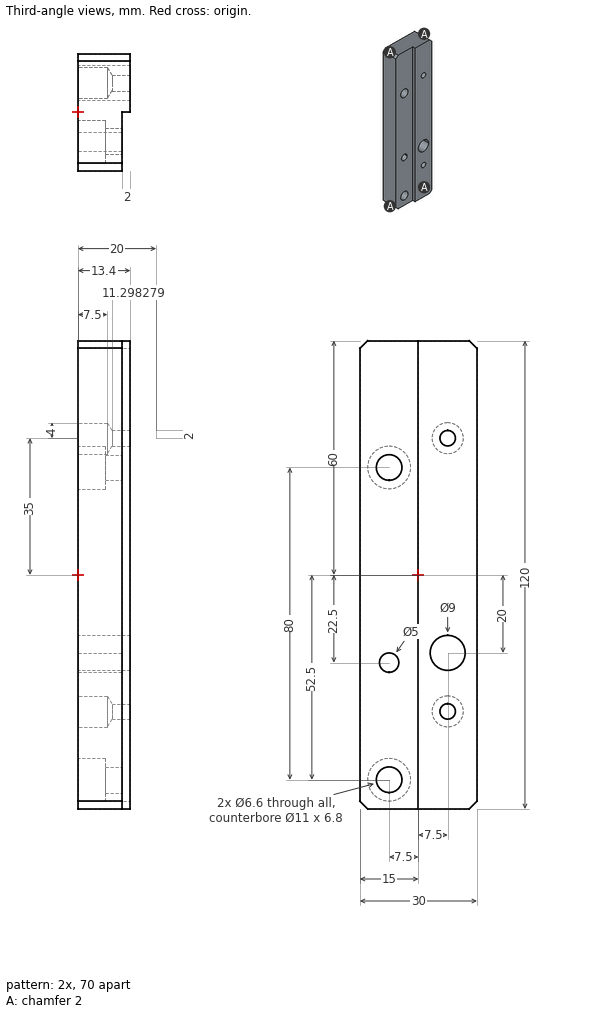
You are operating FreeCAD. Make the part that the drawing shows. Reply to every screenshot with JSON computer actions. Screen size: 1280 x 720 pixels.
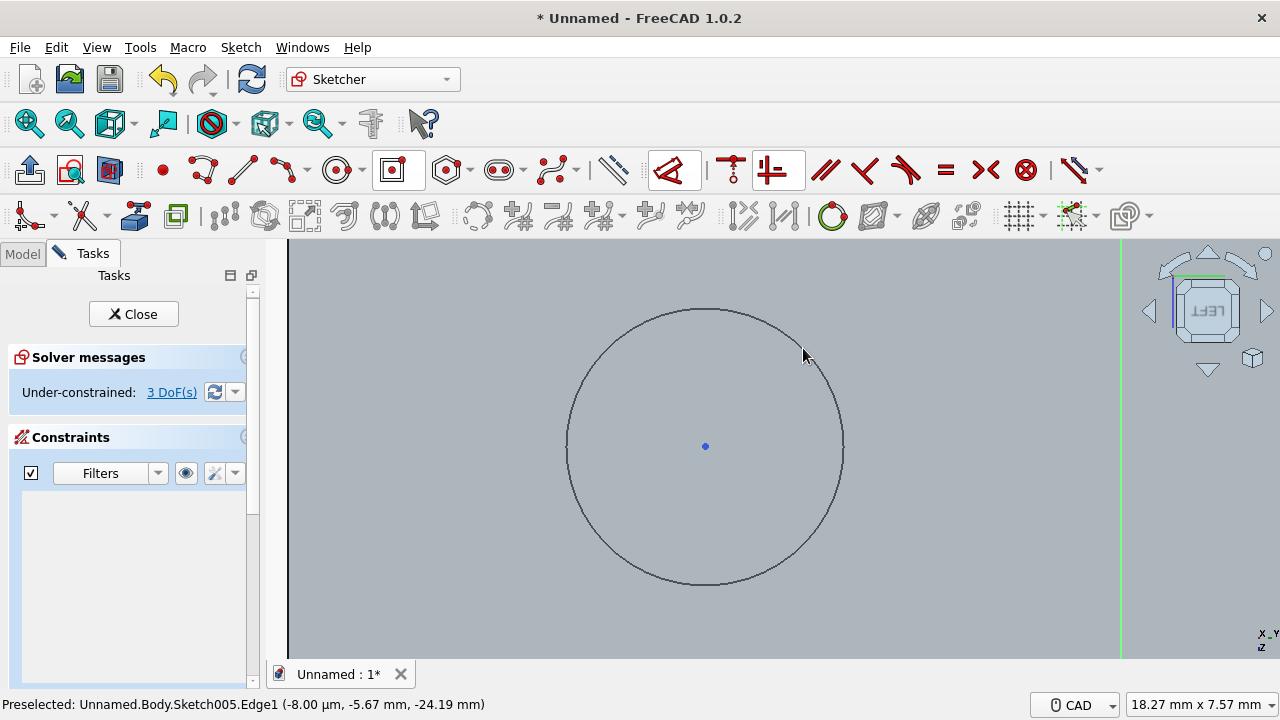
{"action": "left_click", "coordinate": [803, 349]}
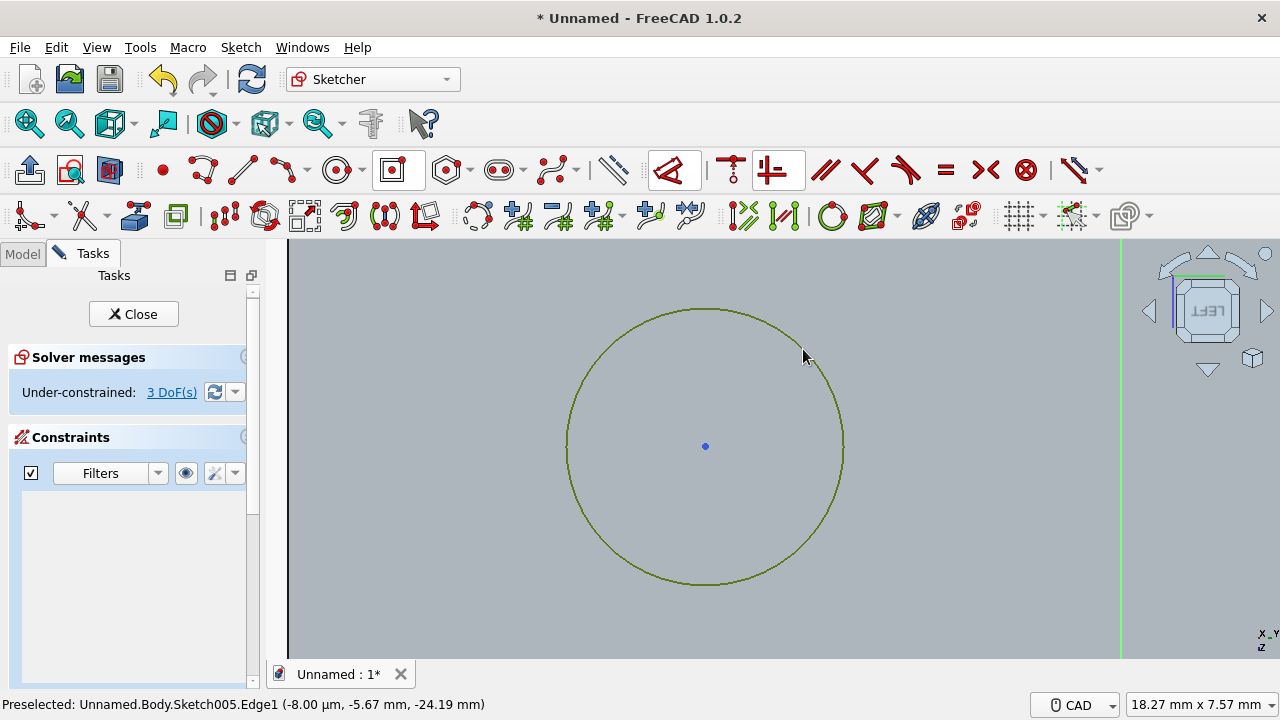
{"action": "left_click", "coordinate": [696, 170]}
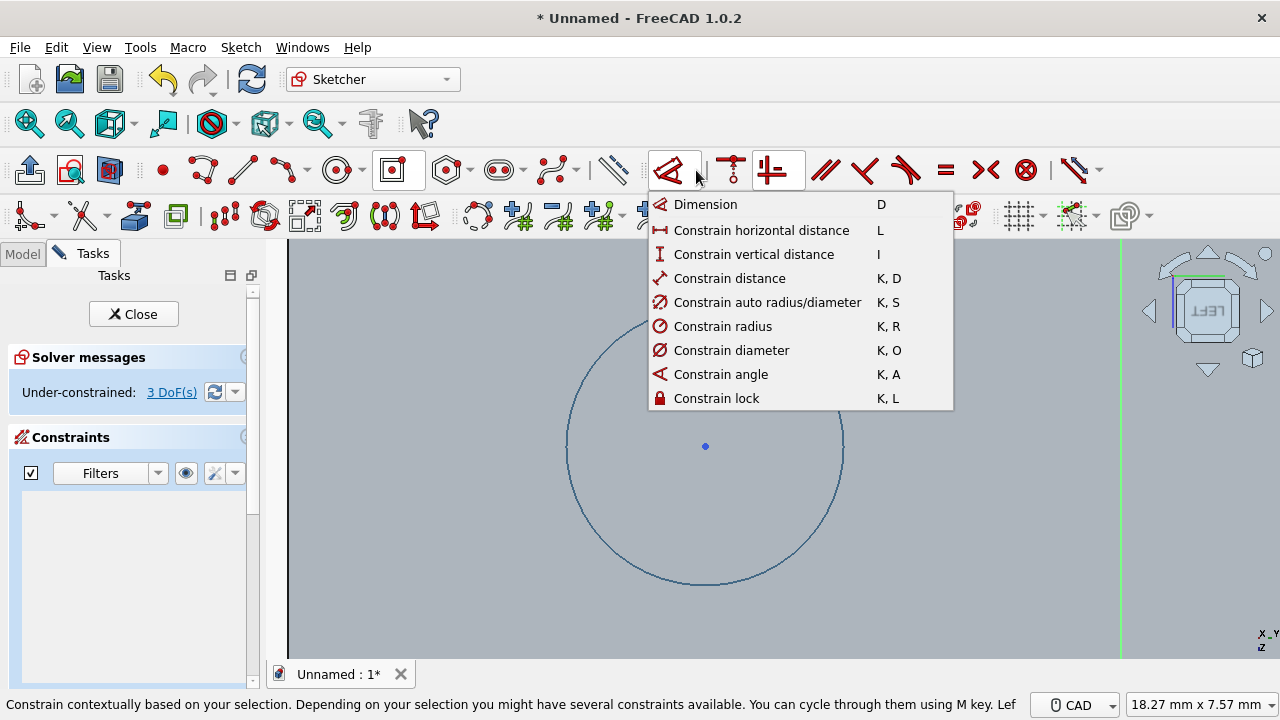
{"action": "left_click", "coordinate": [801, 350]}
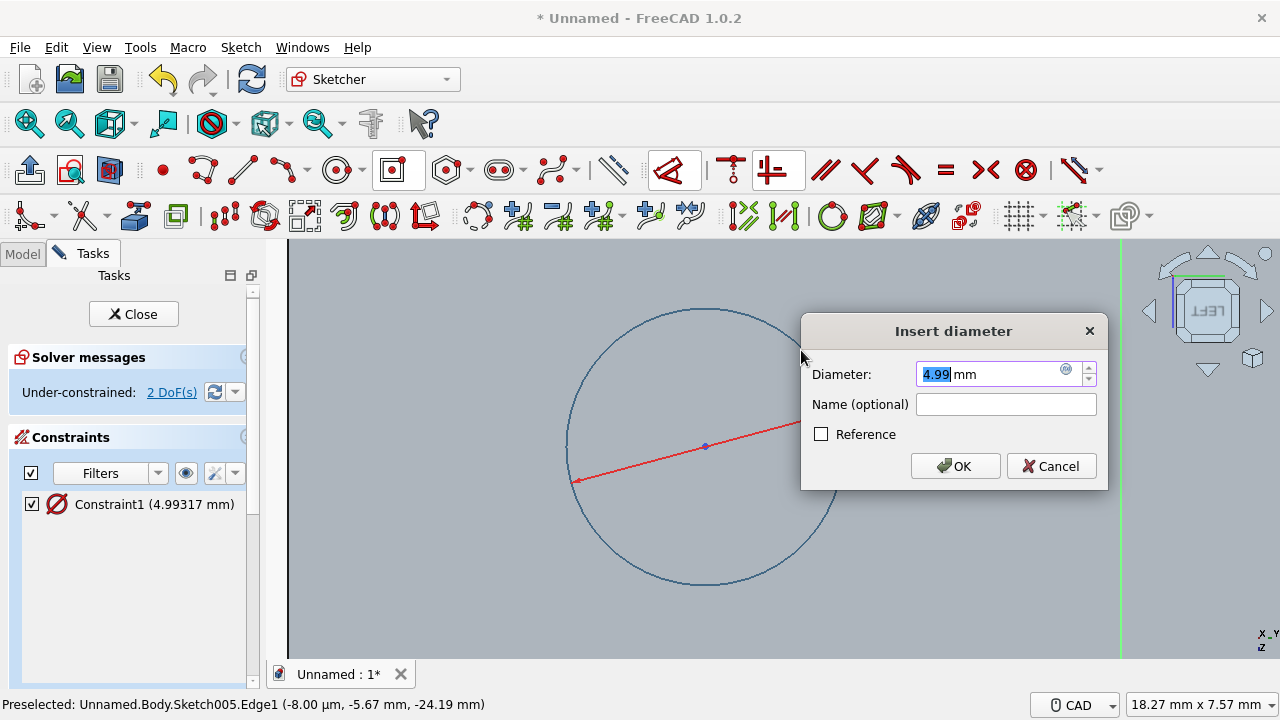
{"action": "type", "text": "5"}
{"action": "key", "text": "Return"}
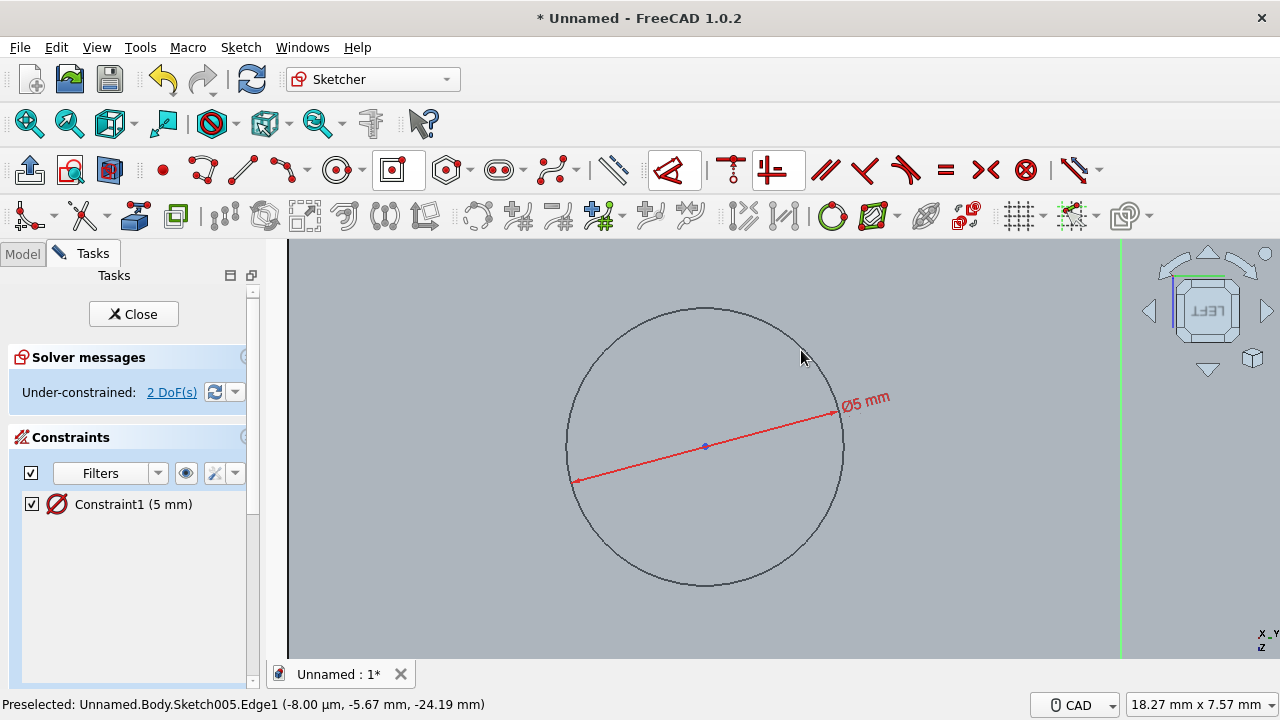
{"action": "left_click", "coordinate": [705, 447]}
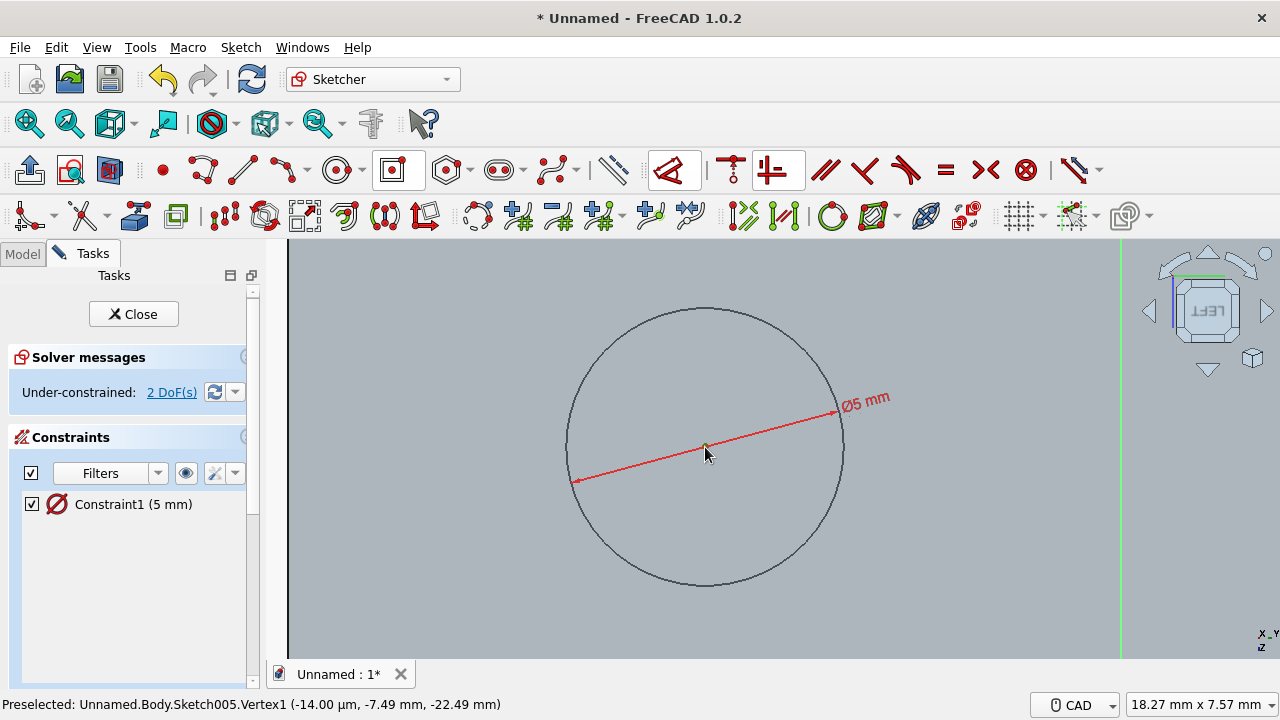
{"action": "key", "text": "l"}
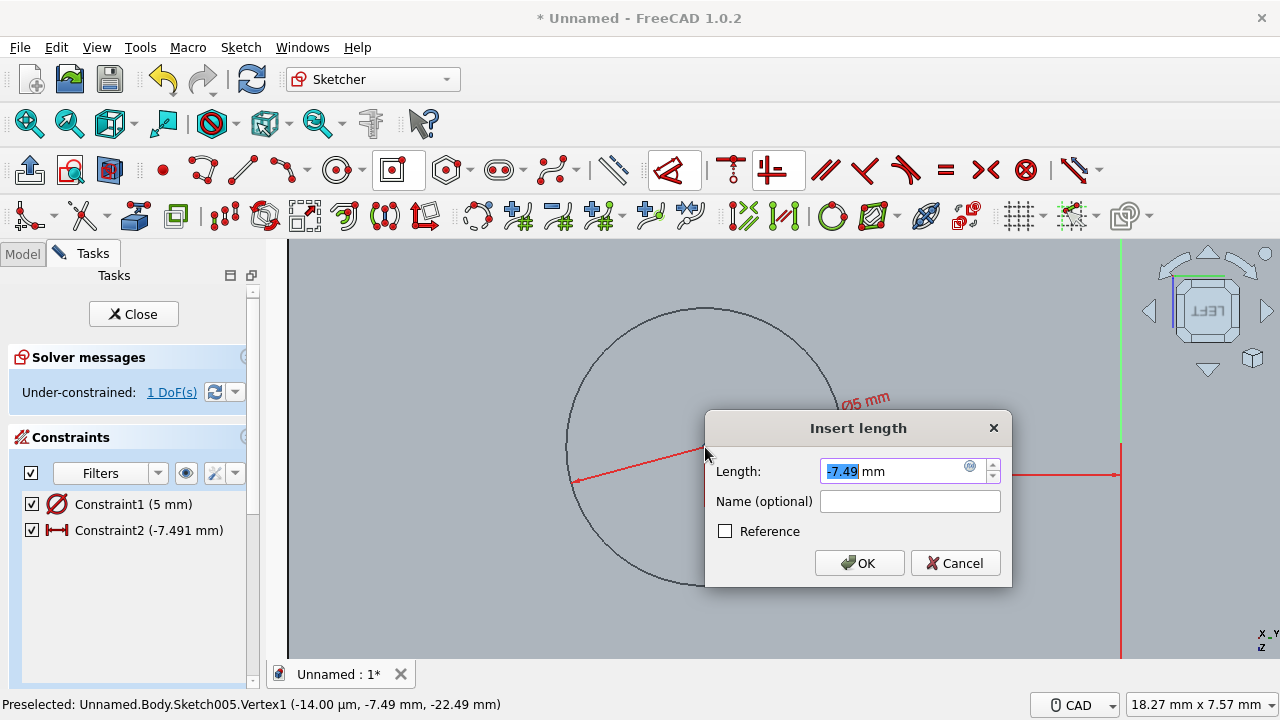
{"action": "type", "text": "-7.5"}
{"action": "key", "text": "Return"}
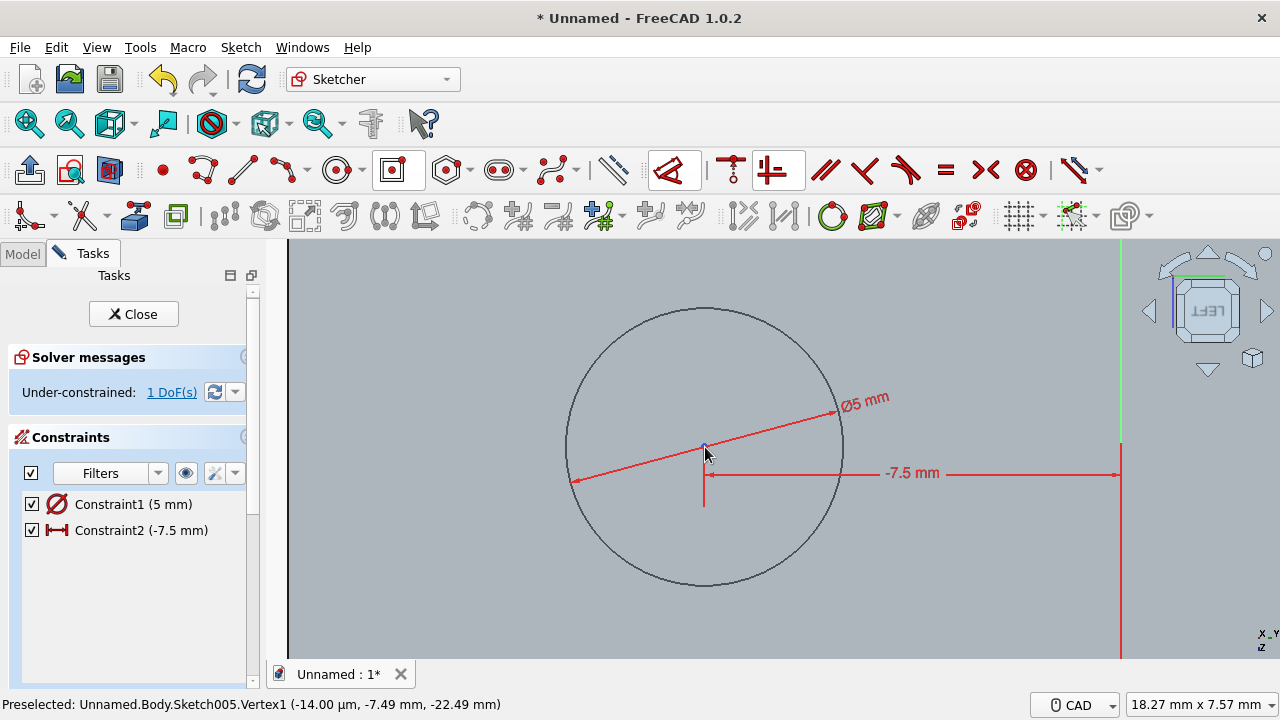
{"action": "left_click", "coordinate": [705, 447]}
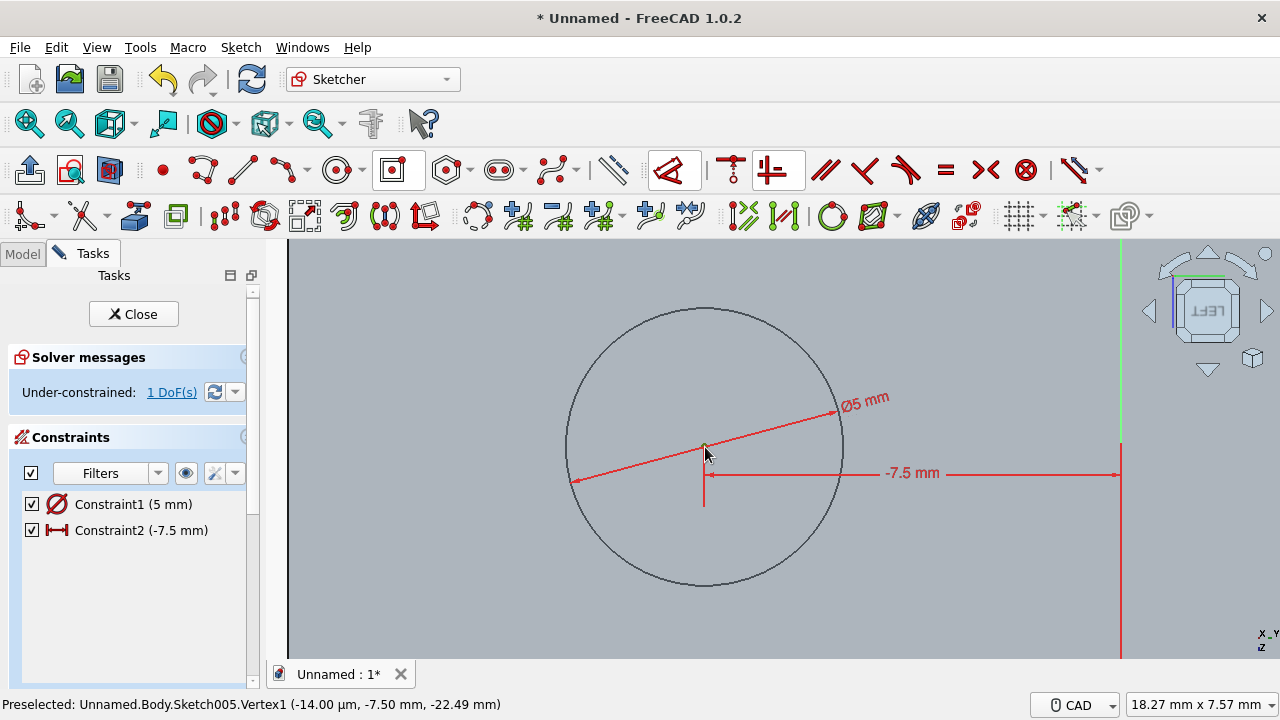
{"action": "key", "text": "i"}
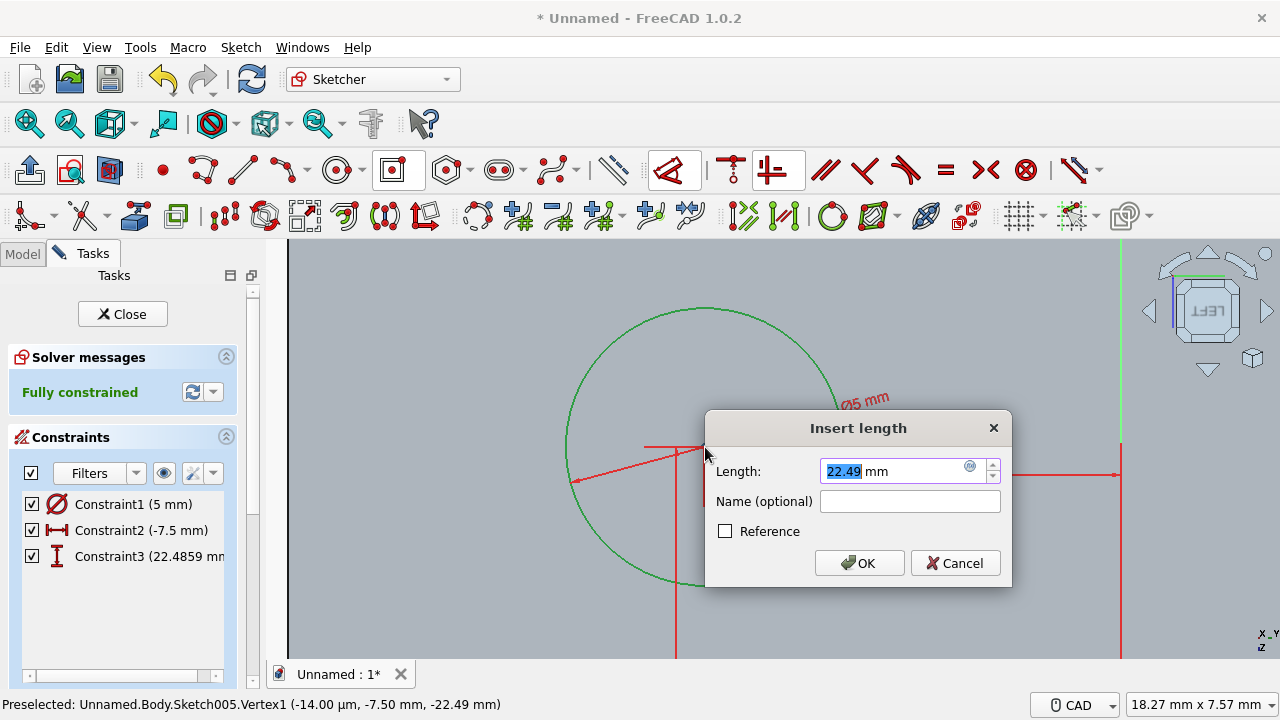
{"action": "type", "text": "22.5"}
{"action": "key", "text": "Return"}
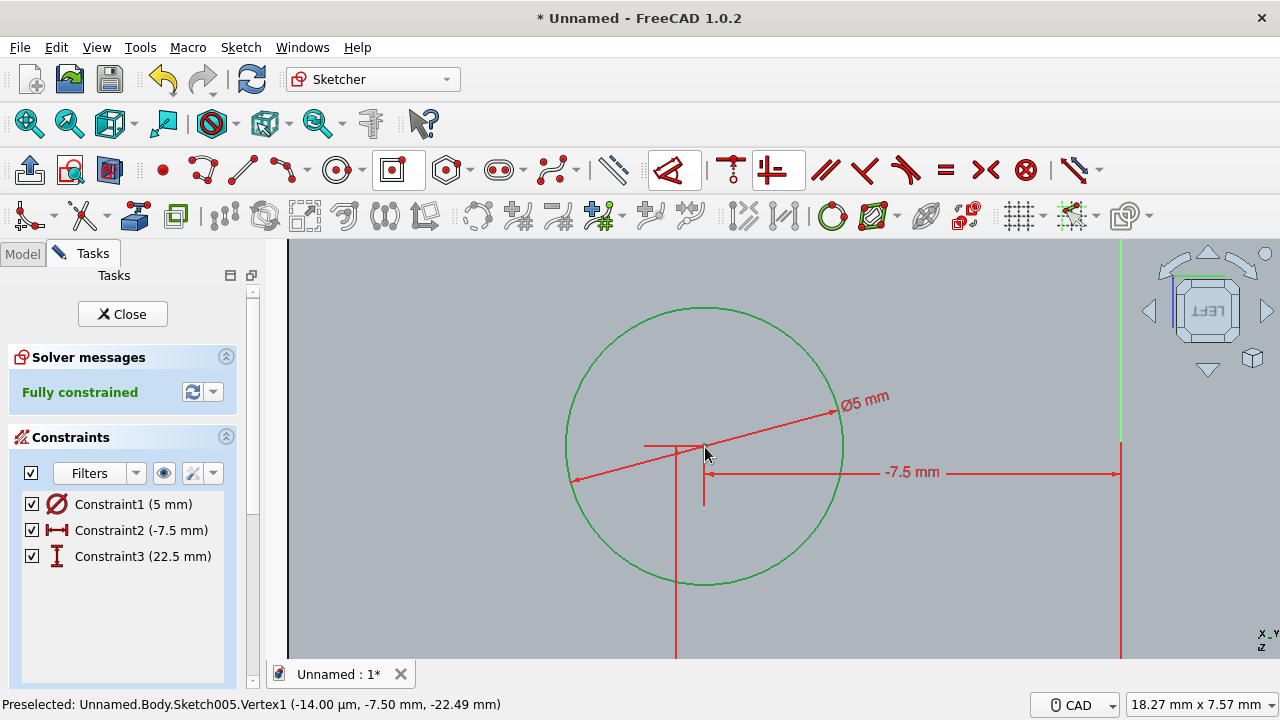
{"action": "left_click", "coordinate": [123, 314]}